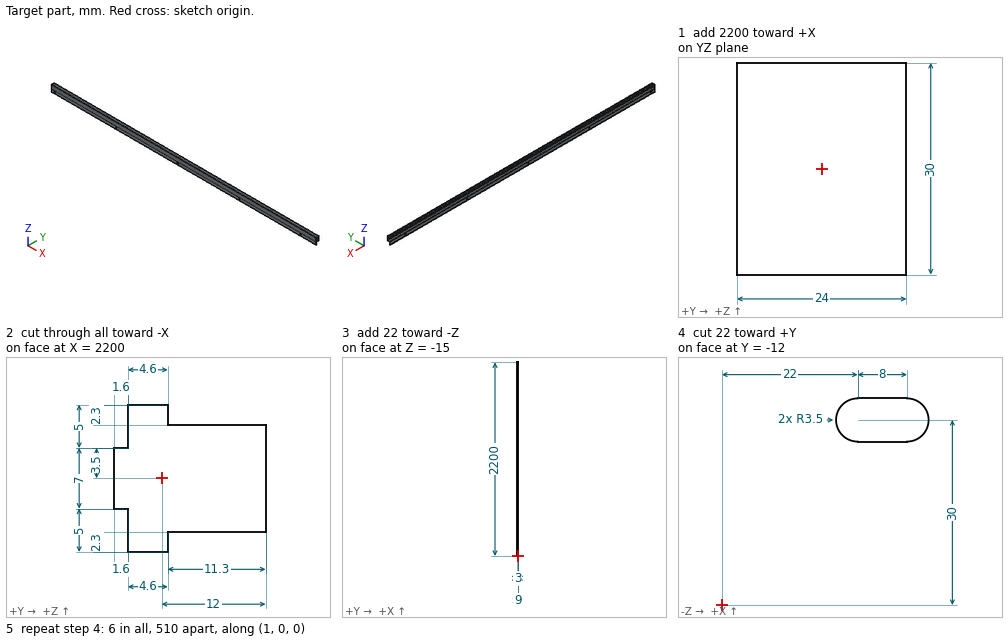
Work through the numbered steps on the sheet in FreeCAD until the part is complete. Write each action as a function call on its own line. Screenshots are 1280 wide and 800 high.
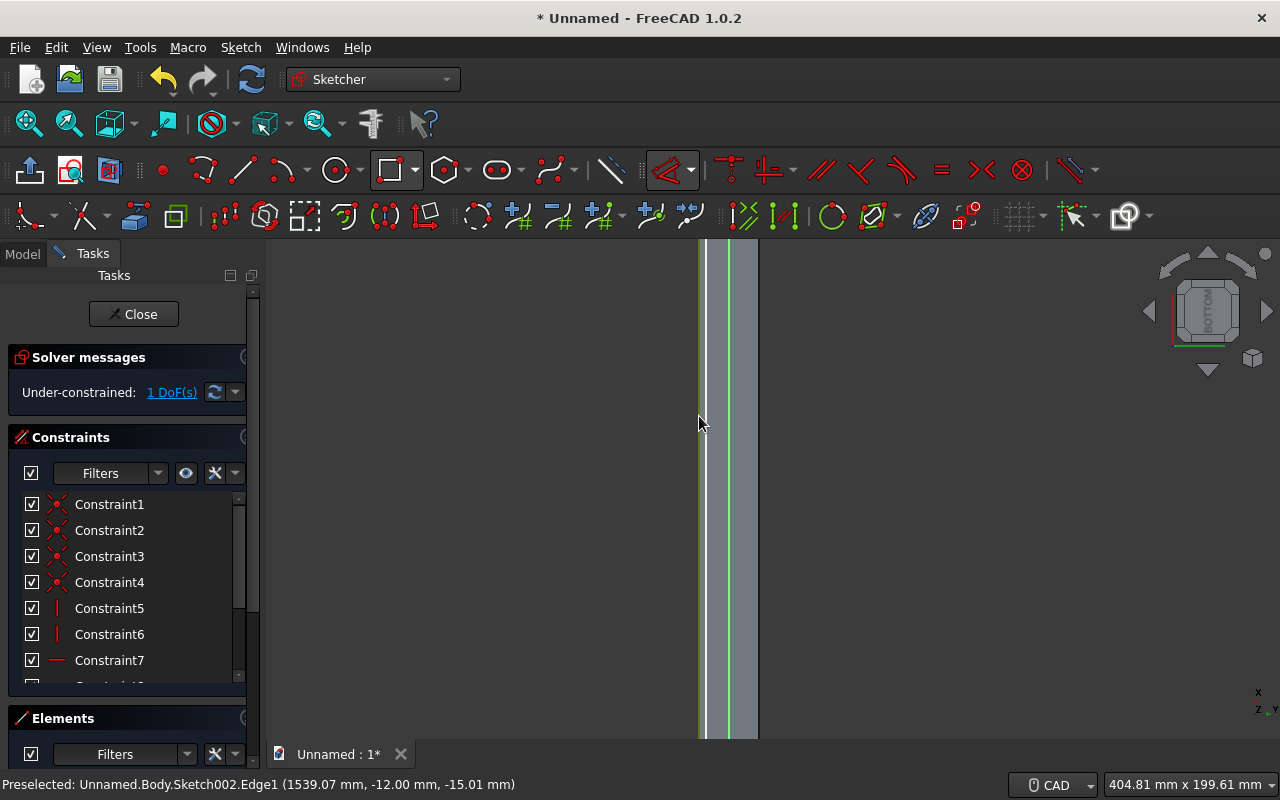
key(i)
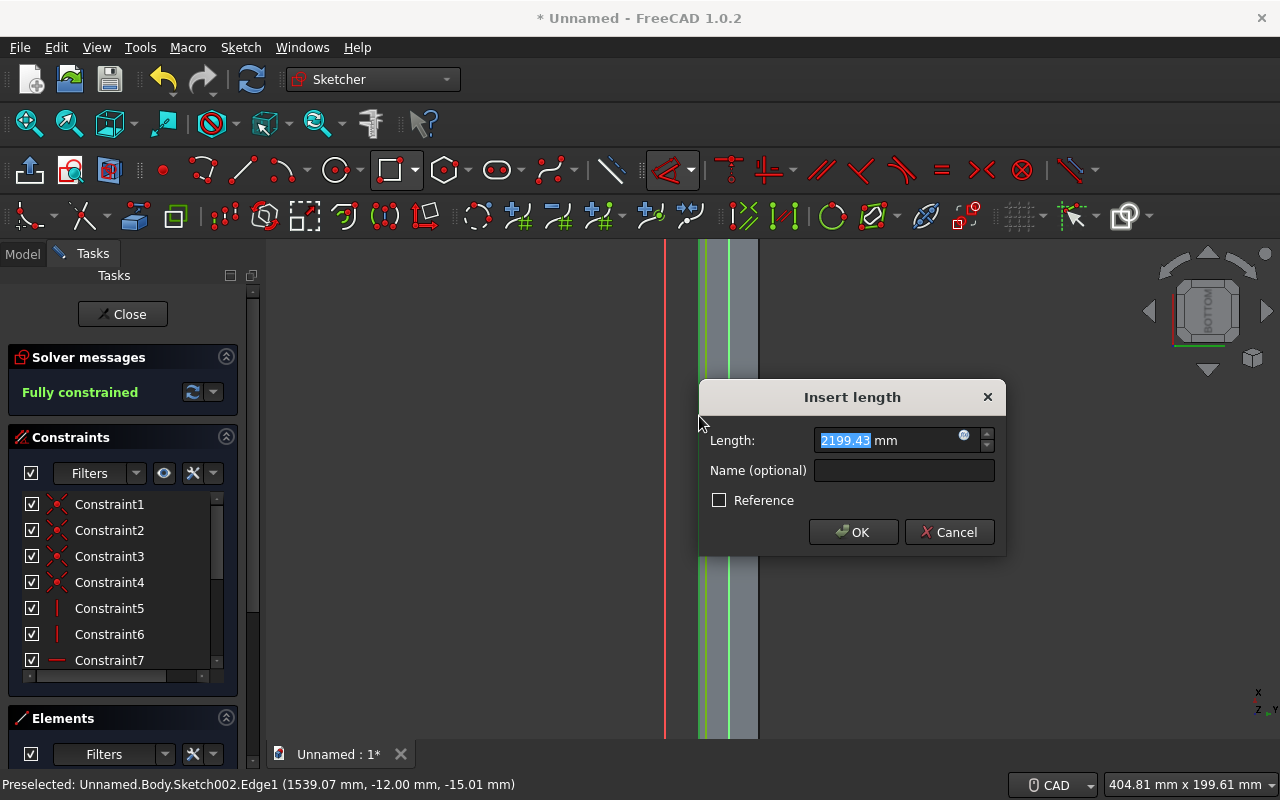
text(2200)
key(Return)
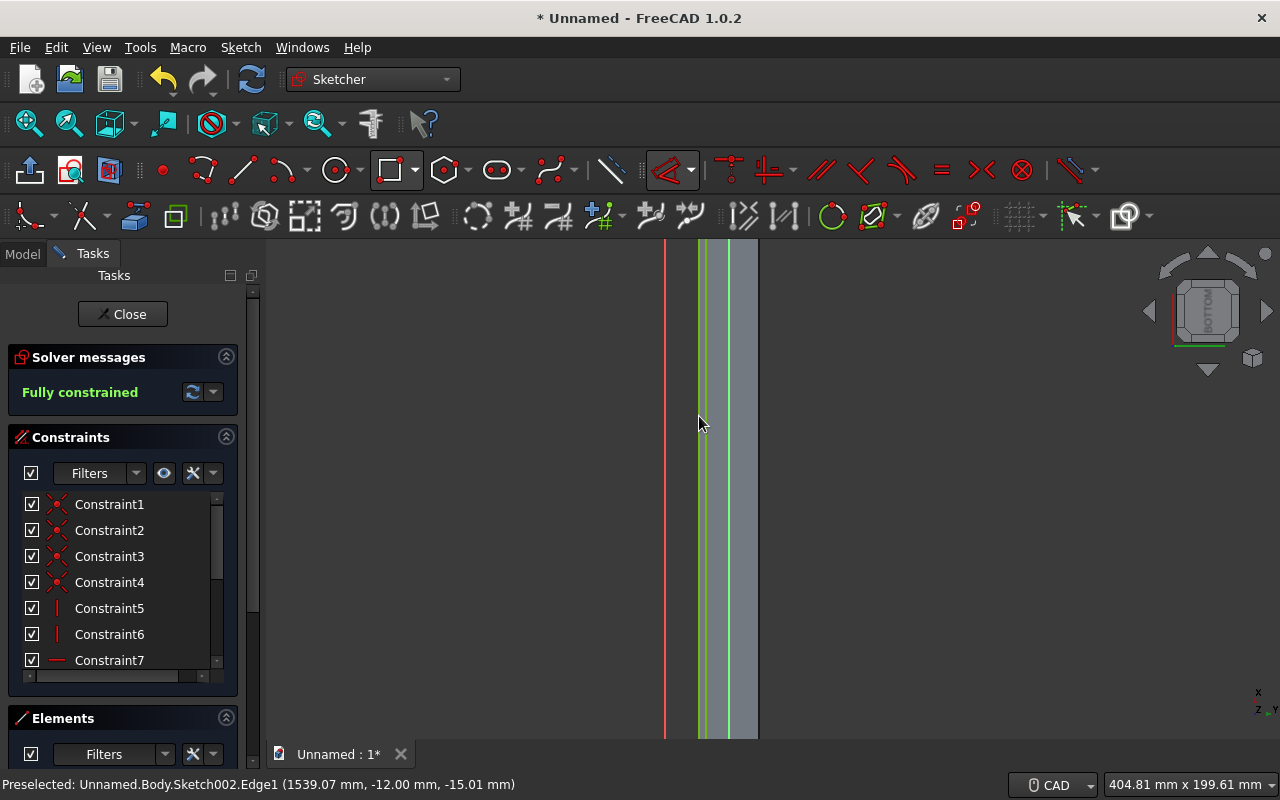
click(123, 314)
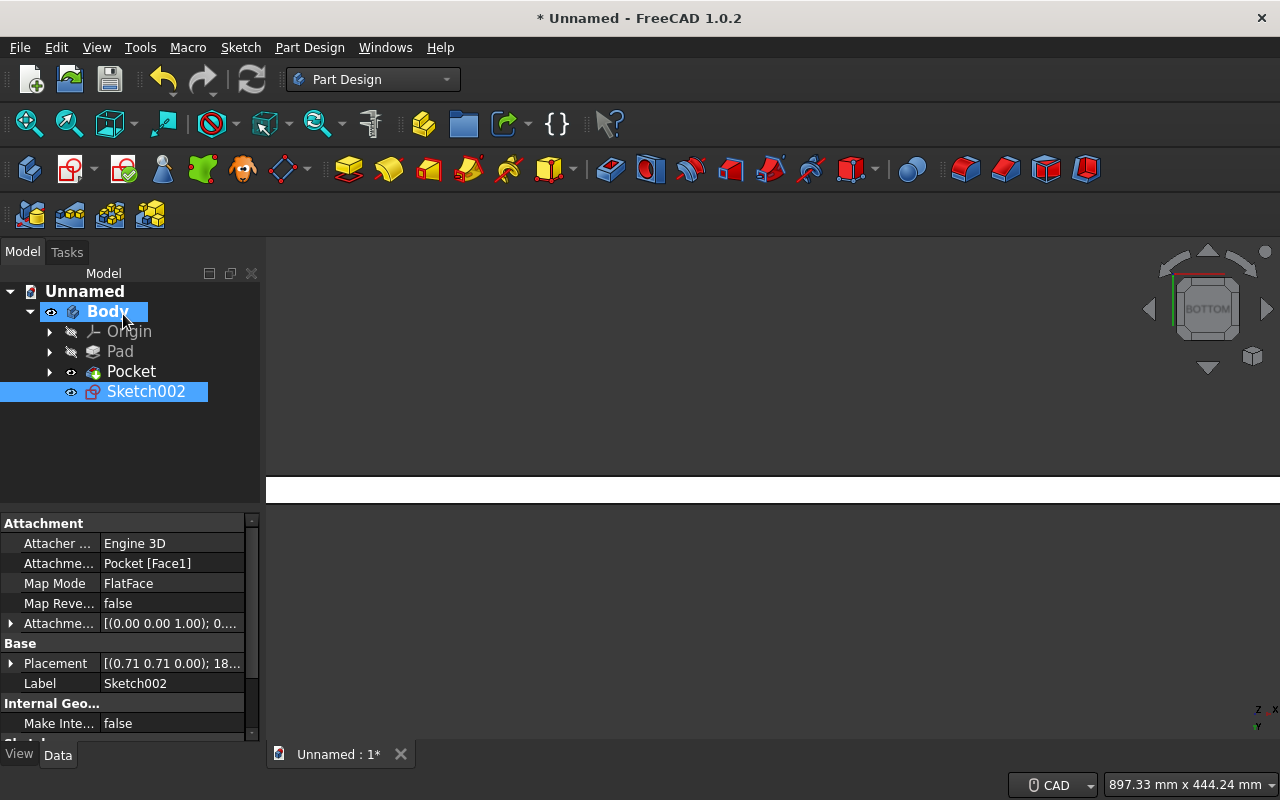
click(350, 170)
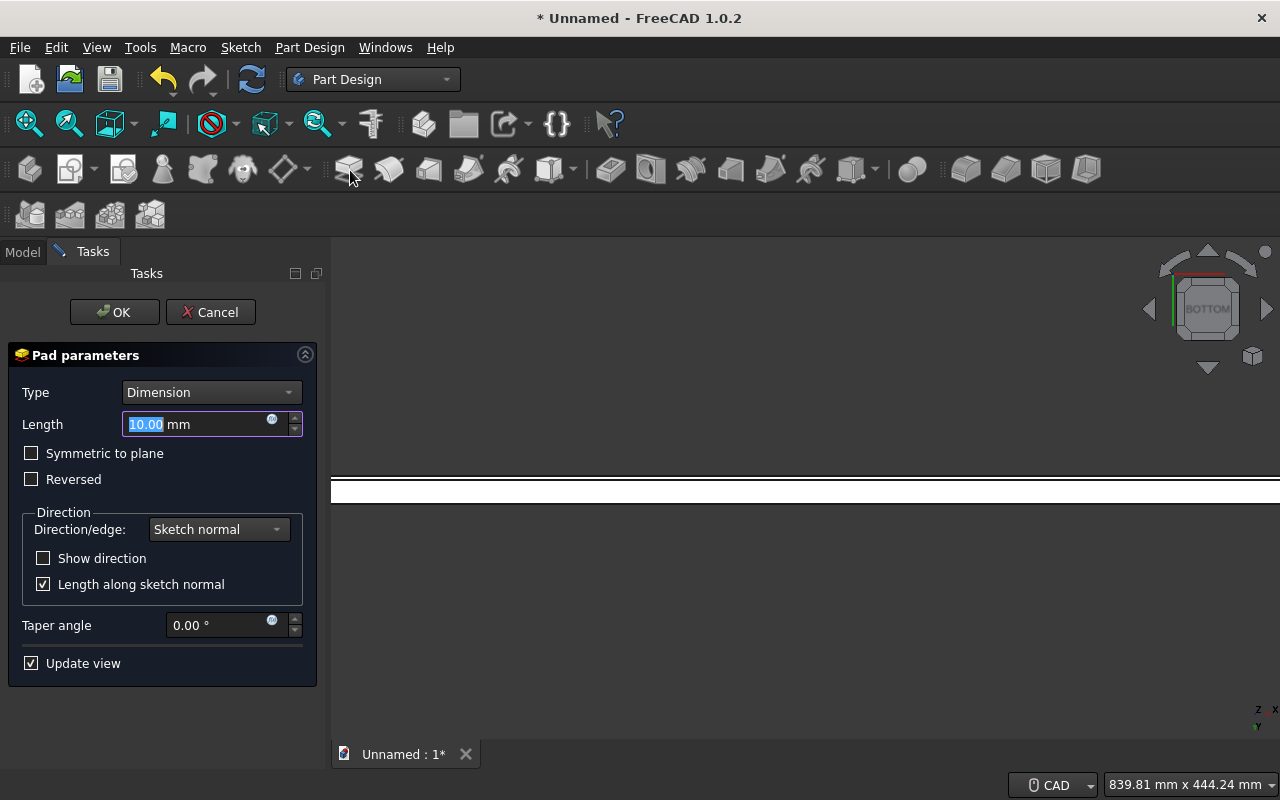
text(22)
key(Tab)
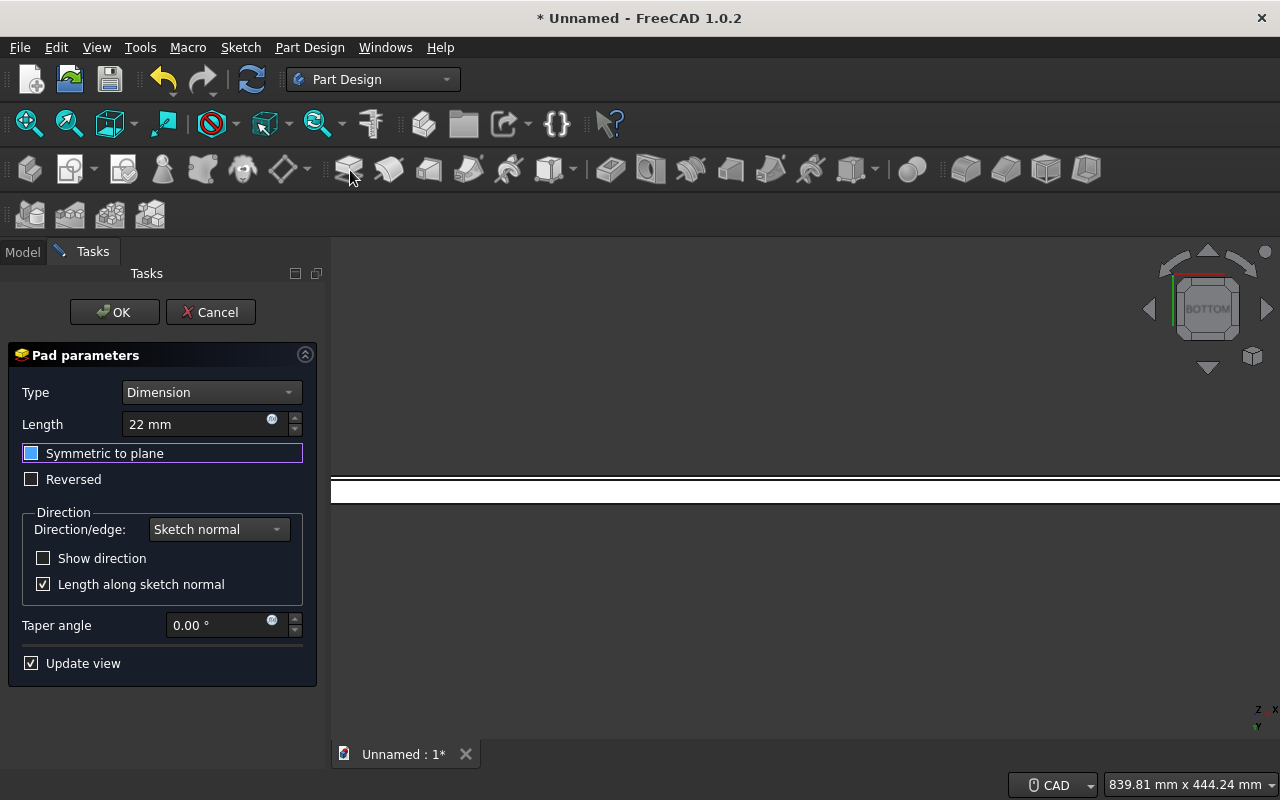
click(115, 312)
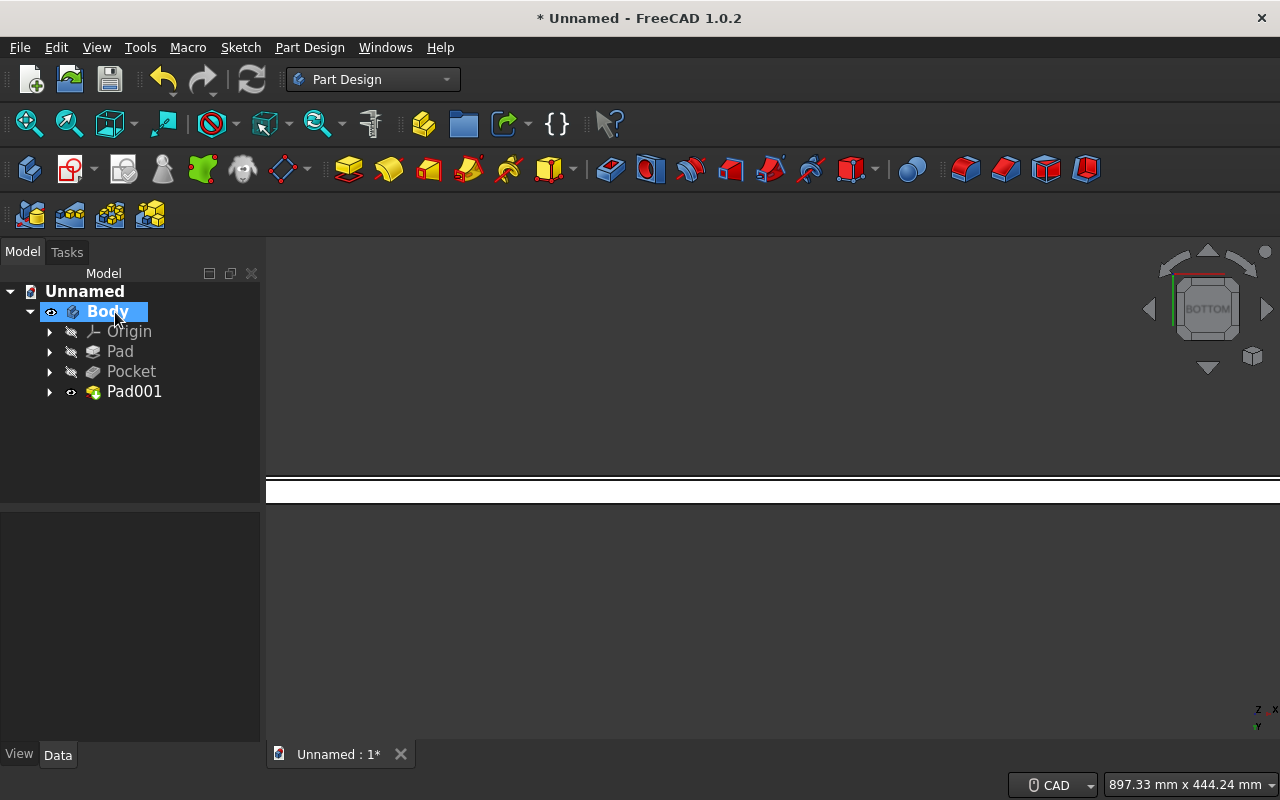
key(v)
key(f)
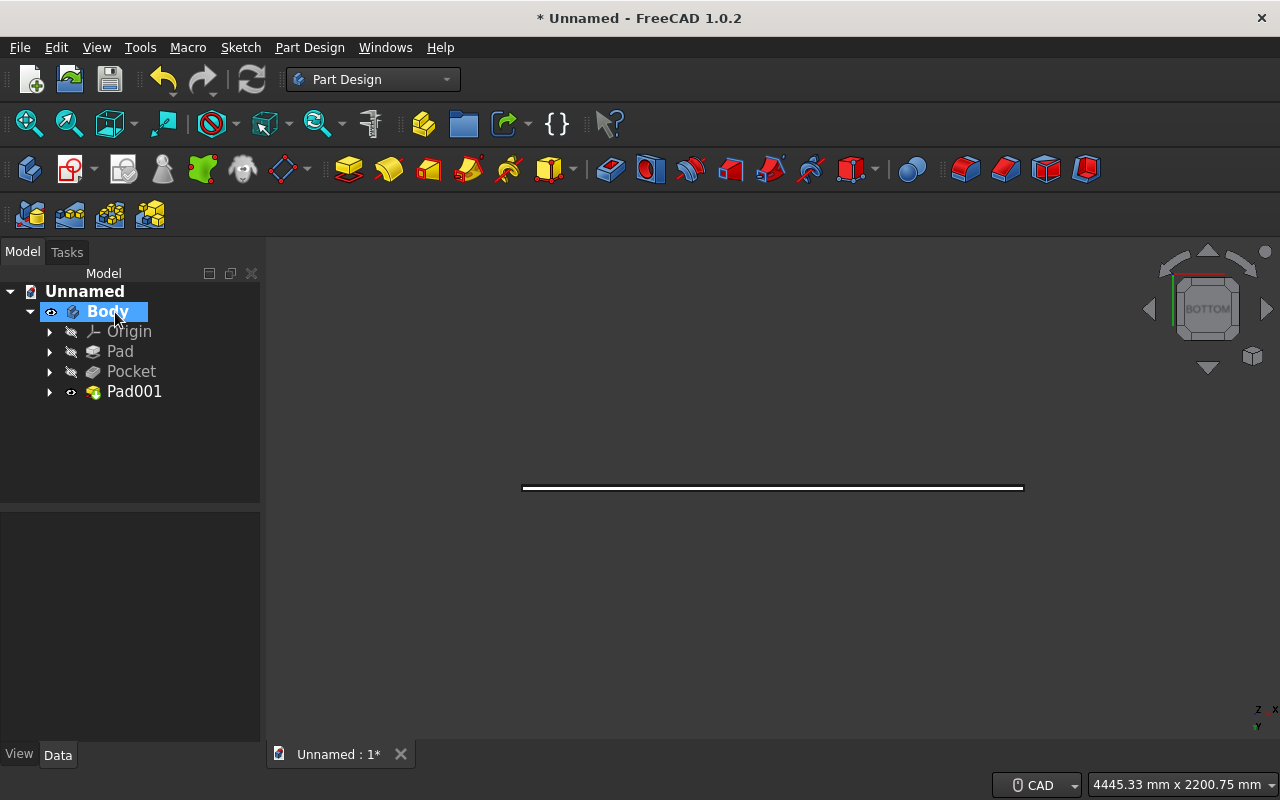
key(0)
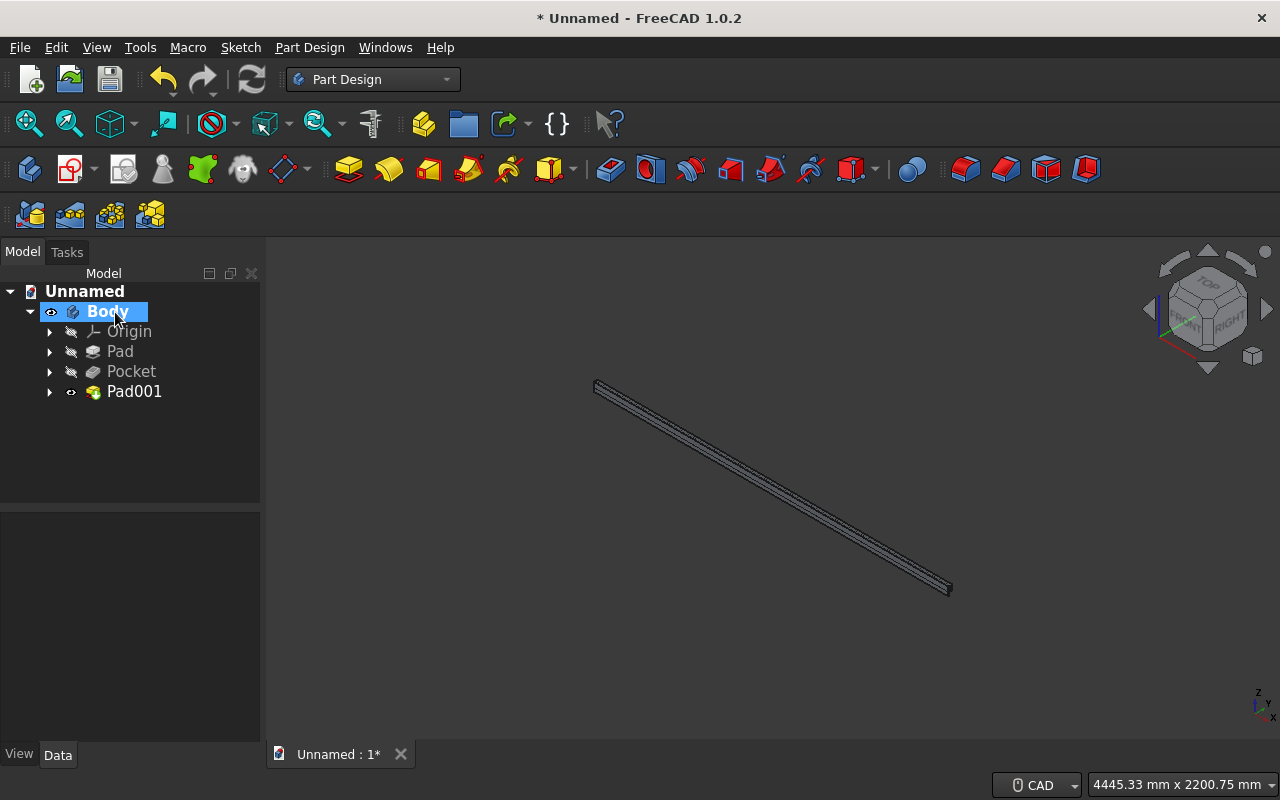
click(30, 124)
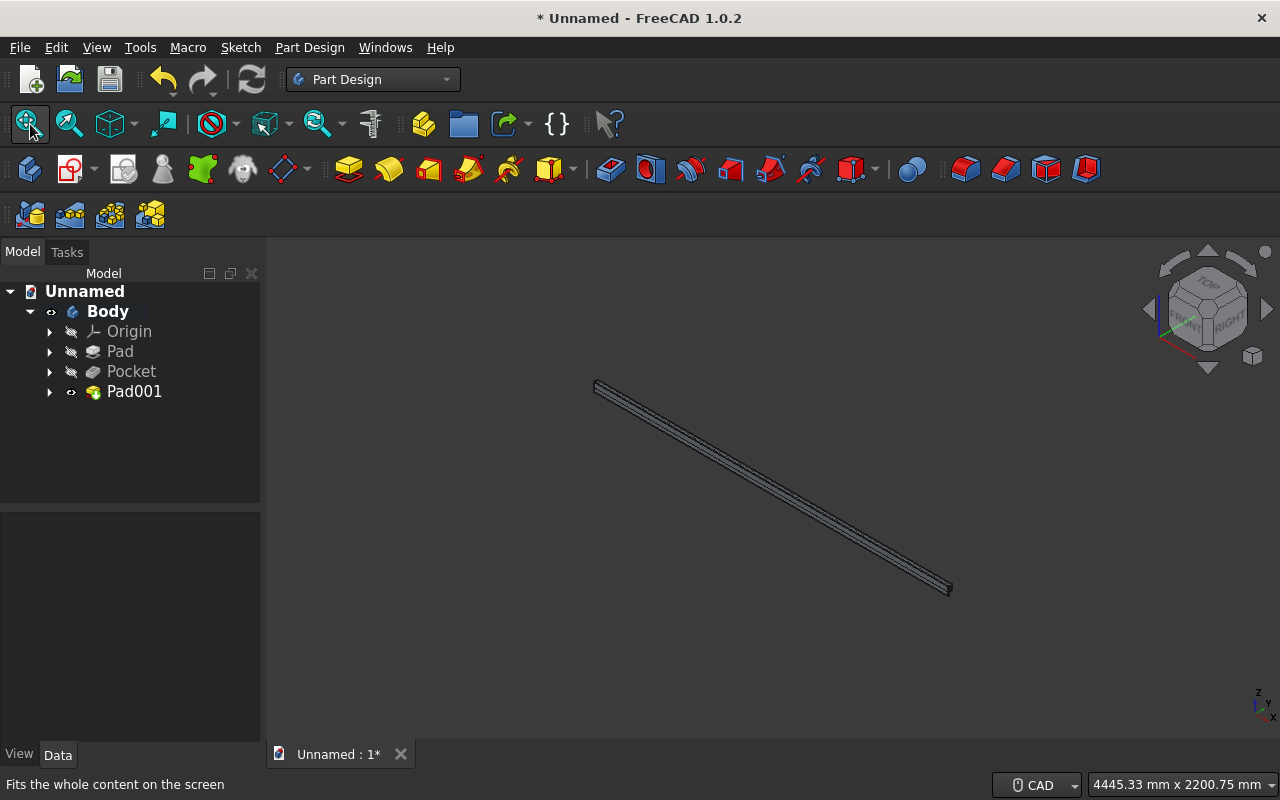
scroll(923, 576, up, 4)